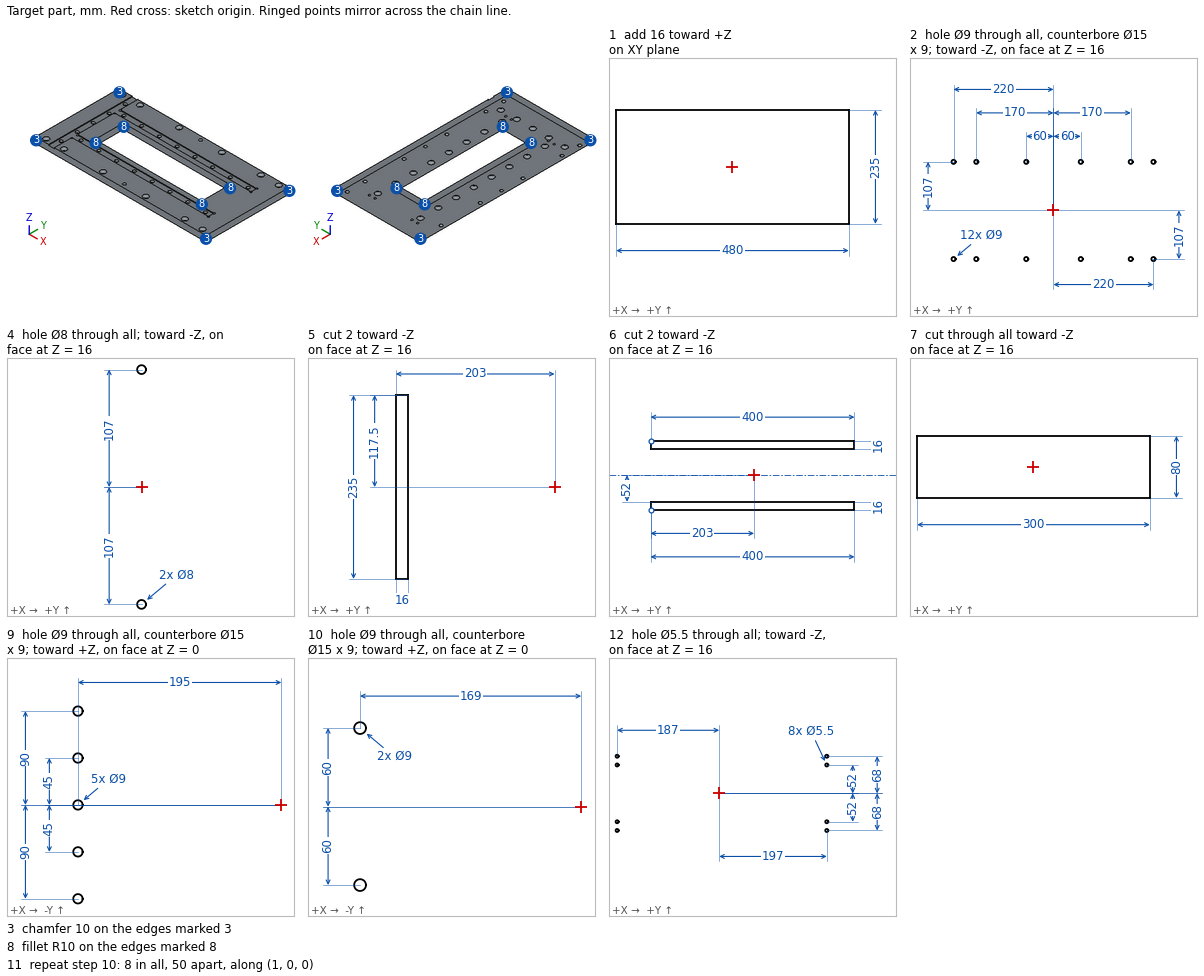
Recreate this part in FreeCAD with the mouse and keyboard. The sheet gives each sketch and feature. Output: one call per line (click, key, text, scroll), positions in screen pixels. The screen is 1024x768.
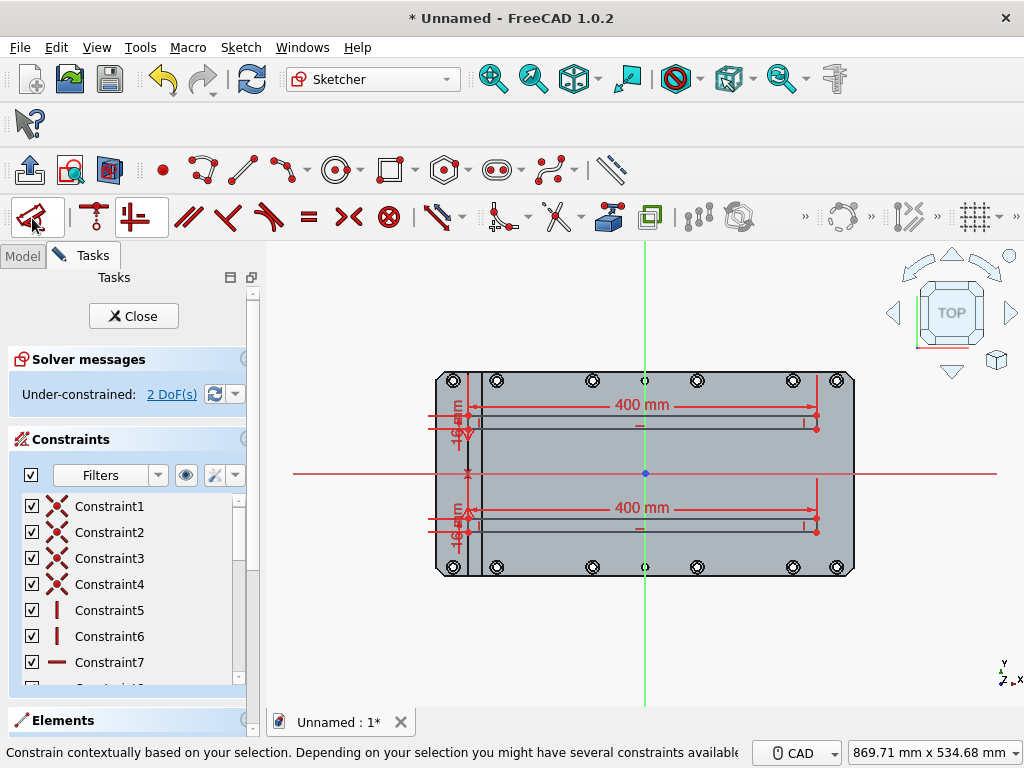
click(468, 519)
click(434, 496)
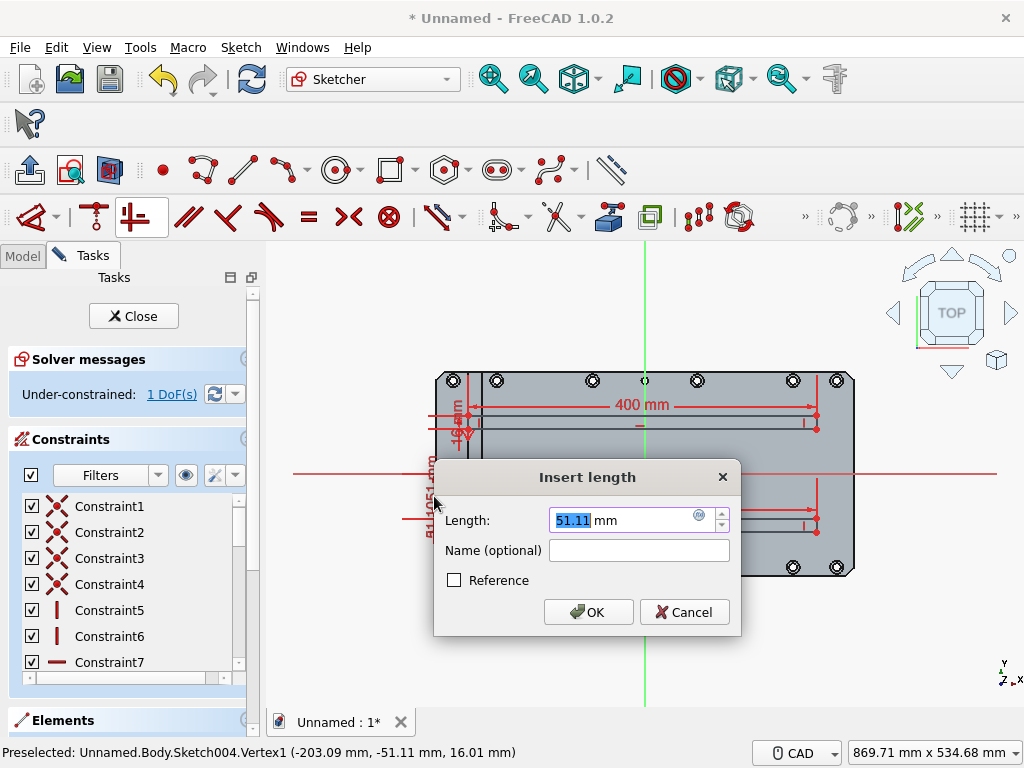
text(52)
key(Return)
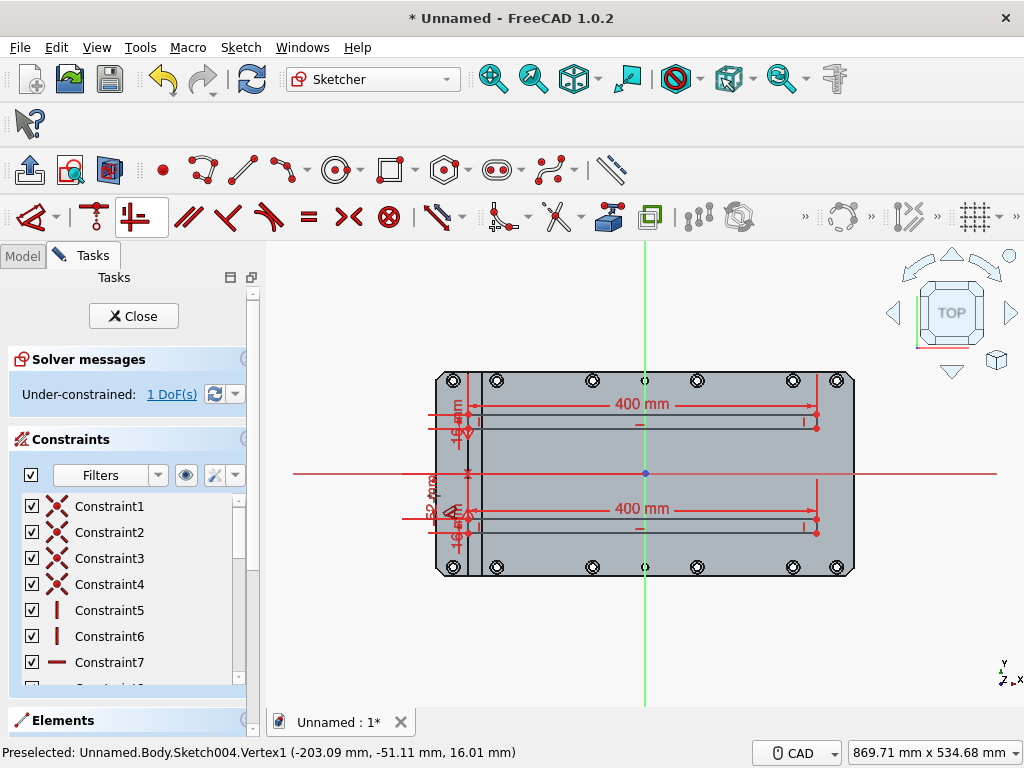
click(468, 519)
click(556, 553)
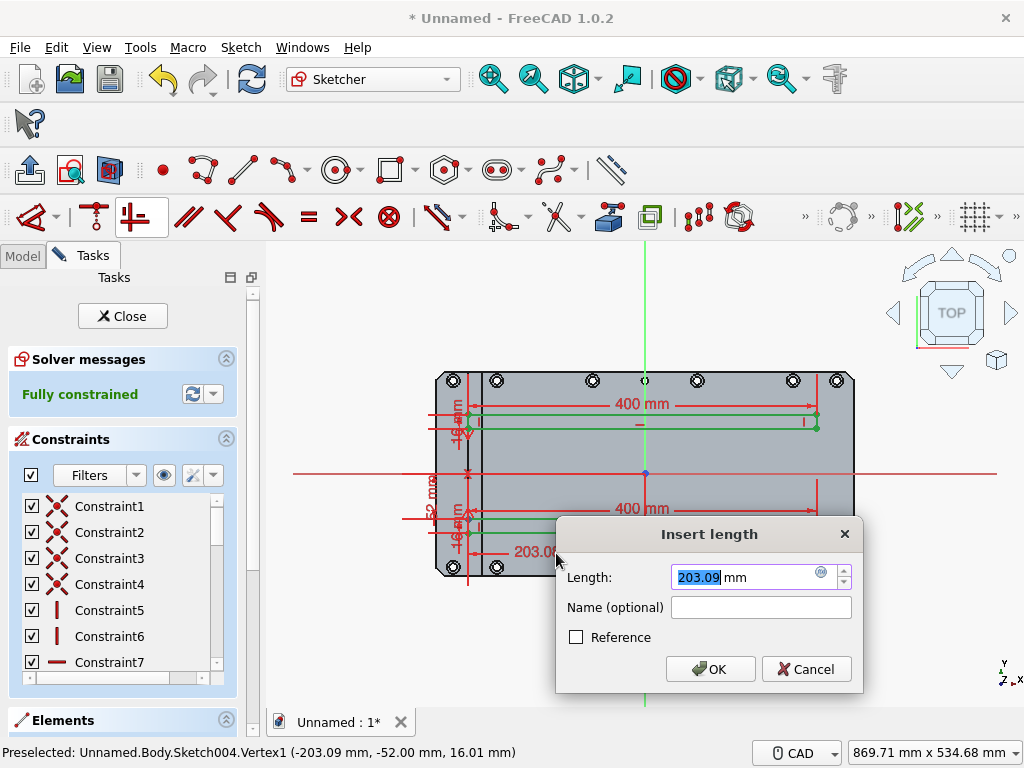
text(203)
key(Return)
key(Escape)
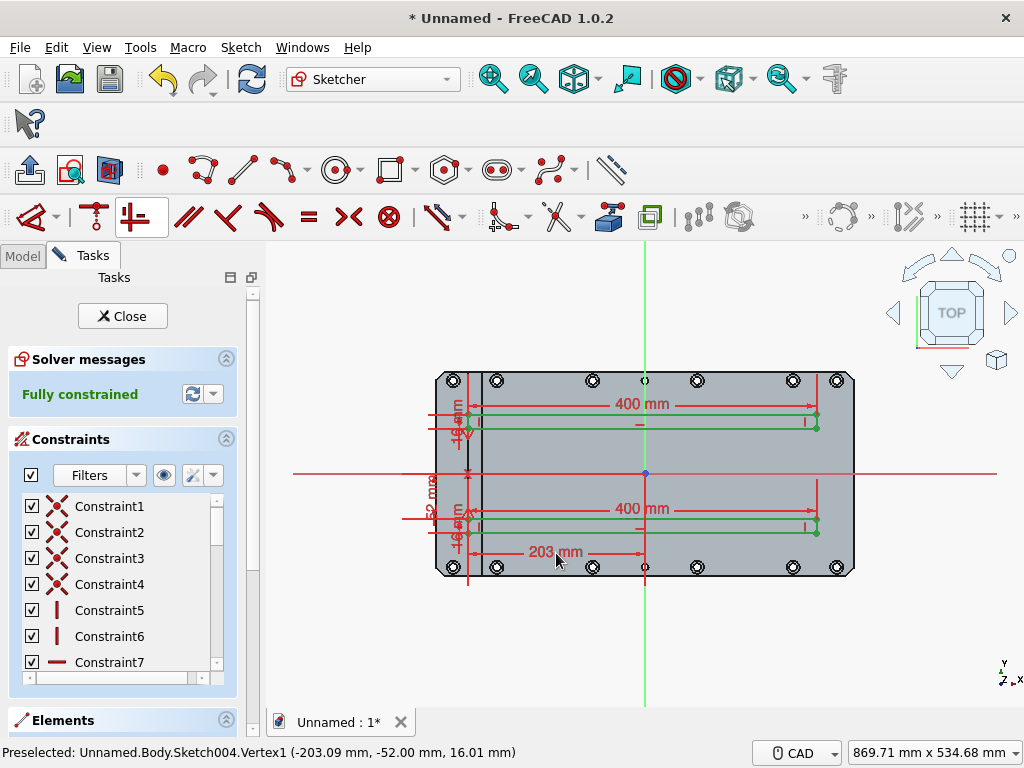
click(123, 316)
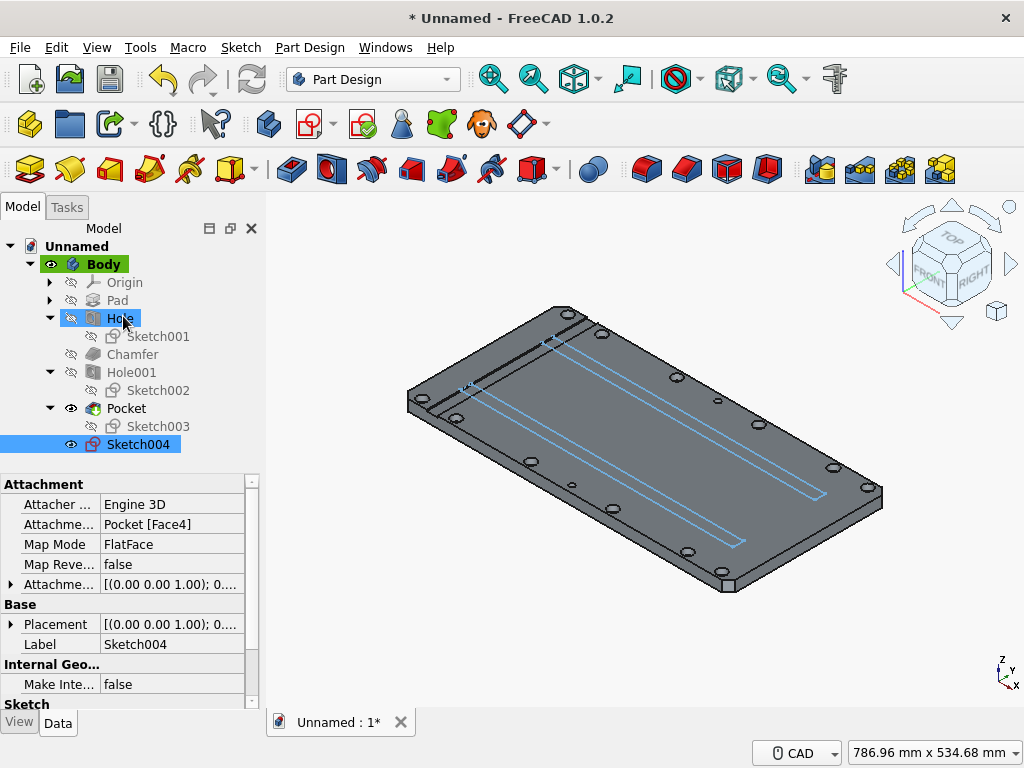
click(292, 170)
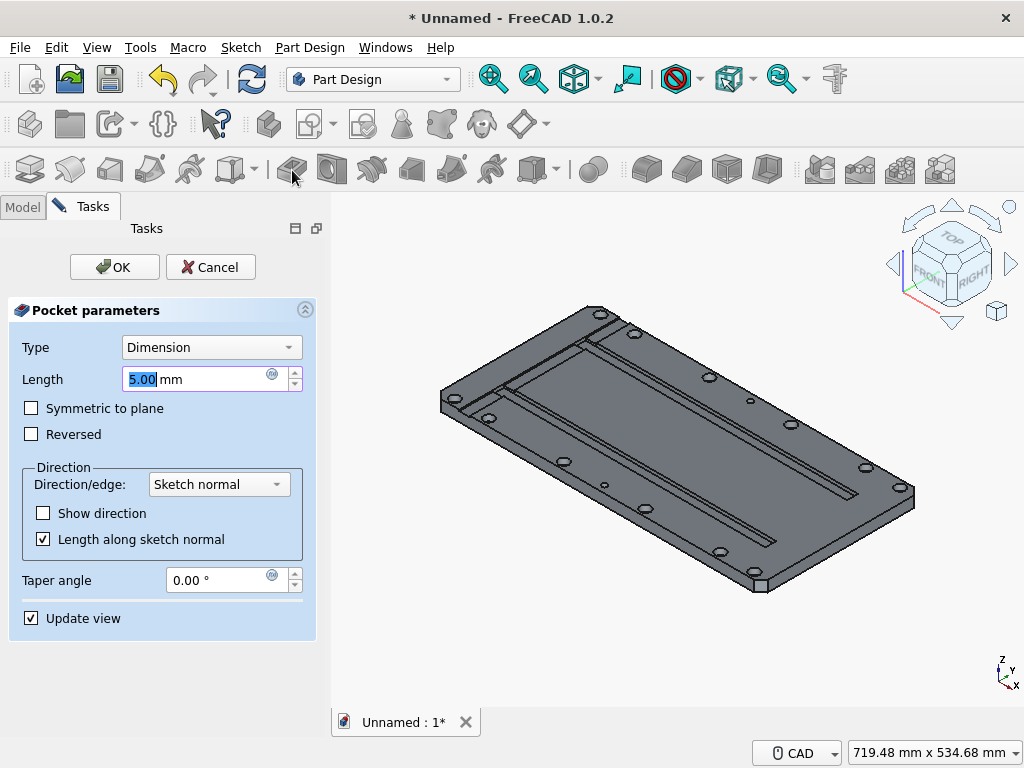
text(2)
key(Tab)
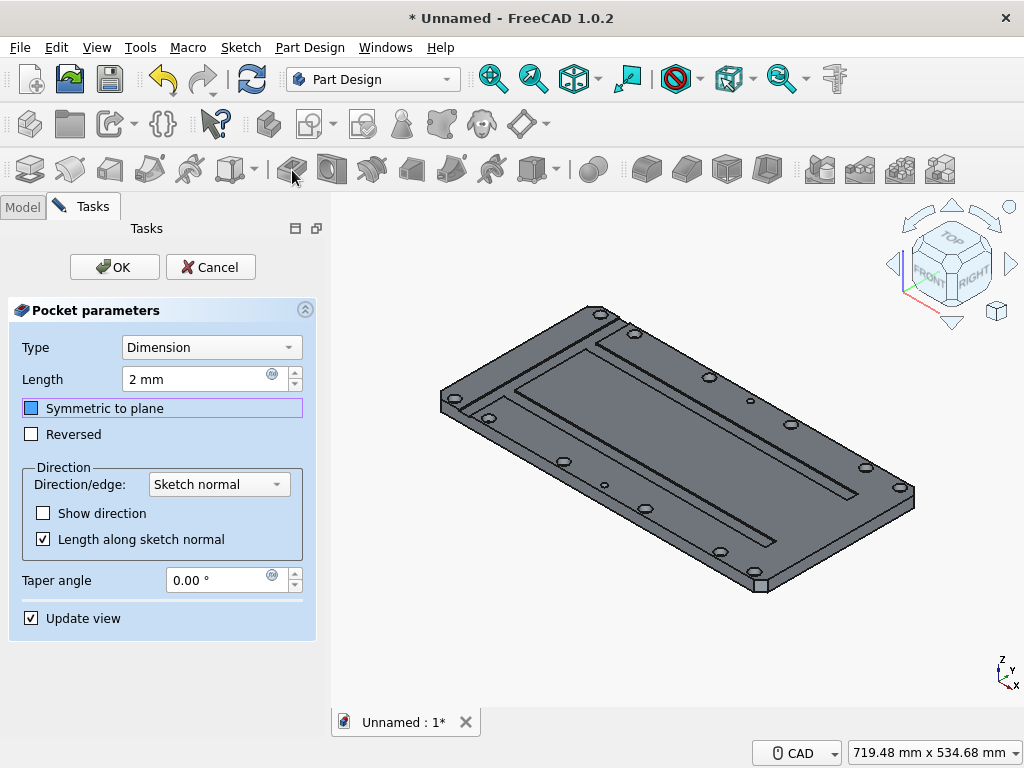
click(115, 267)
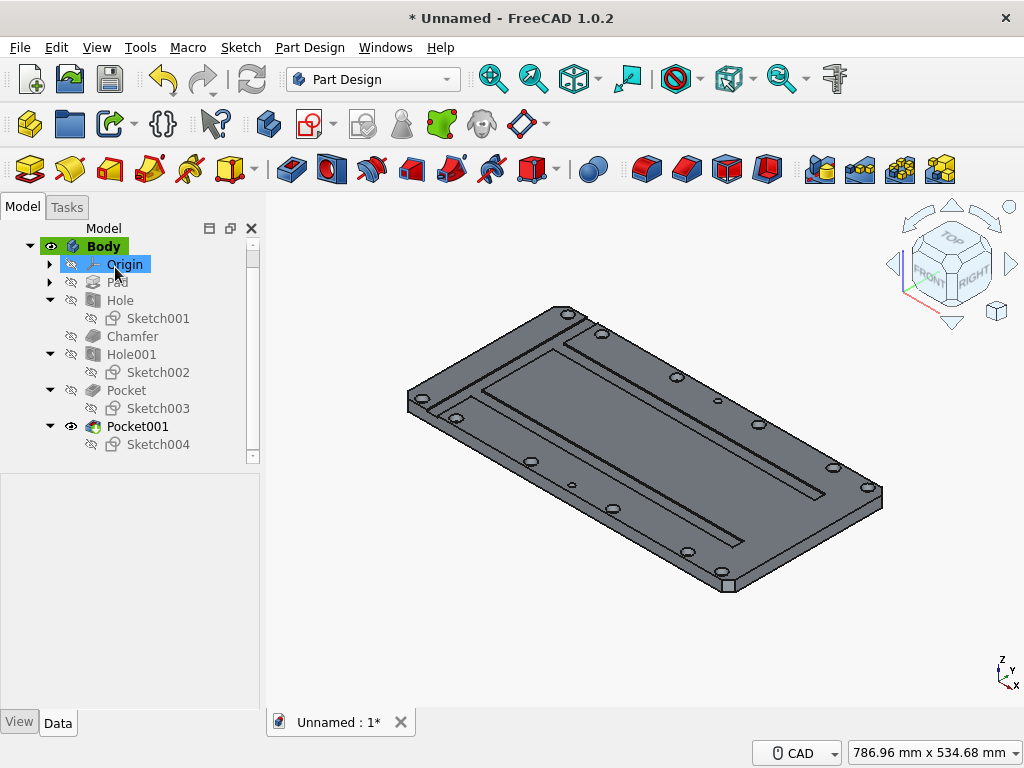
click(746, 501)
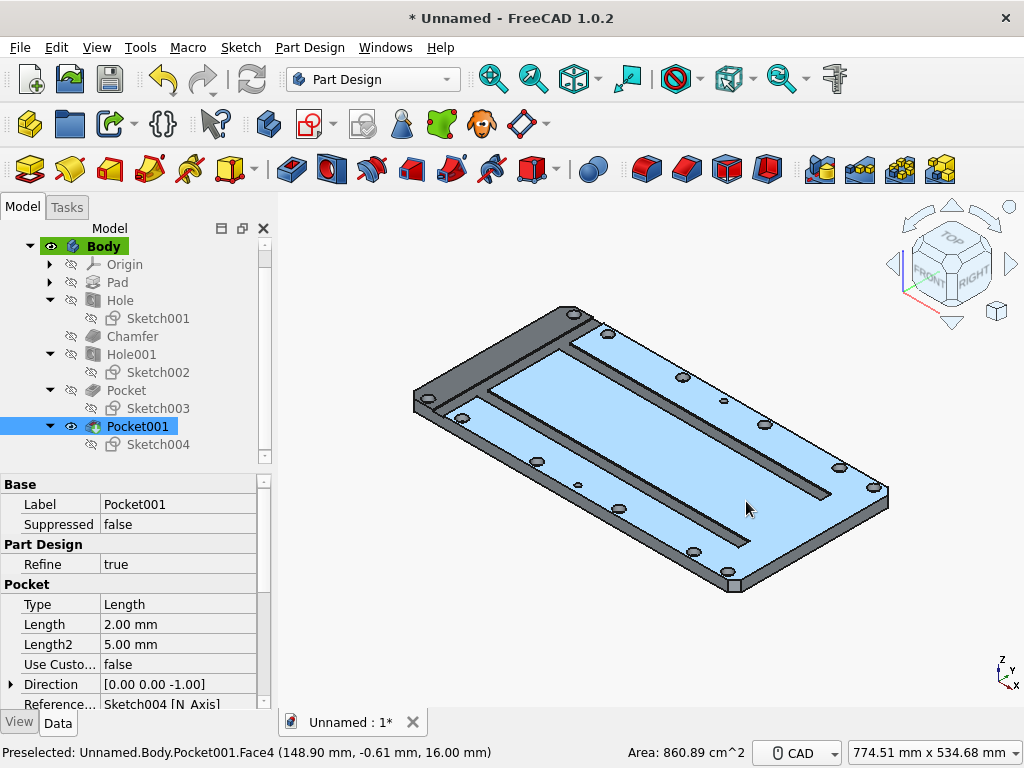
click(310, 124)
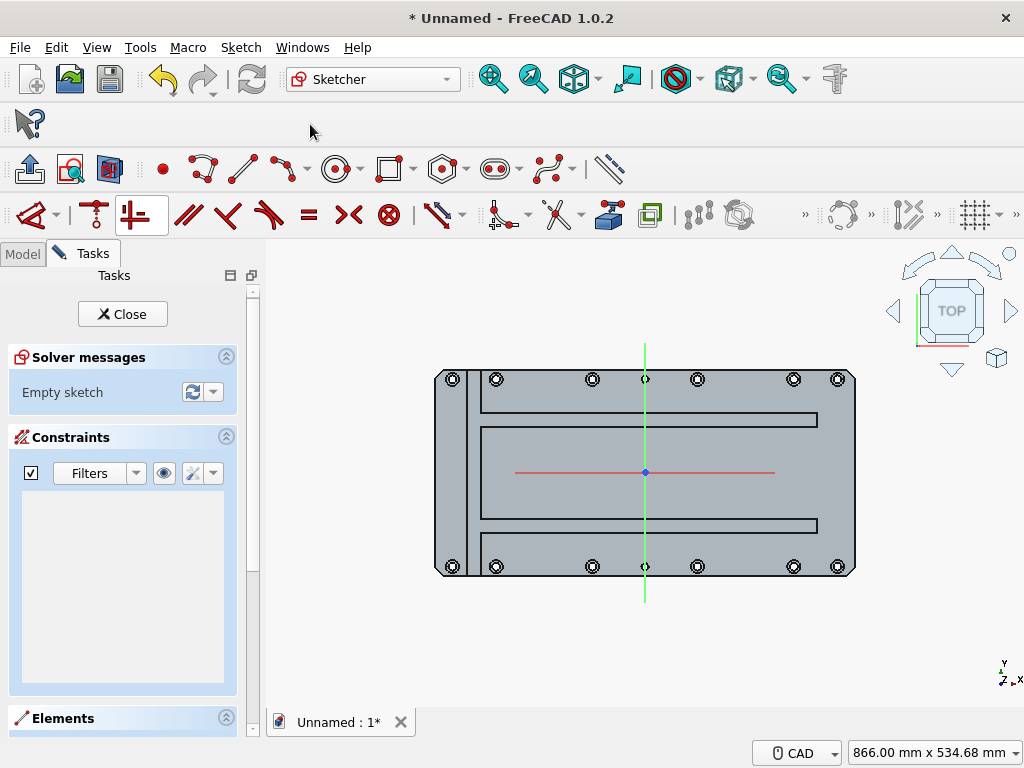
scroll(784, 473, up, 2)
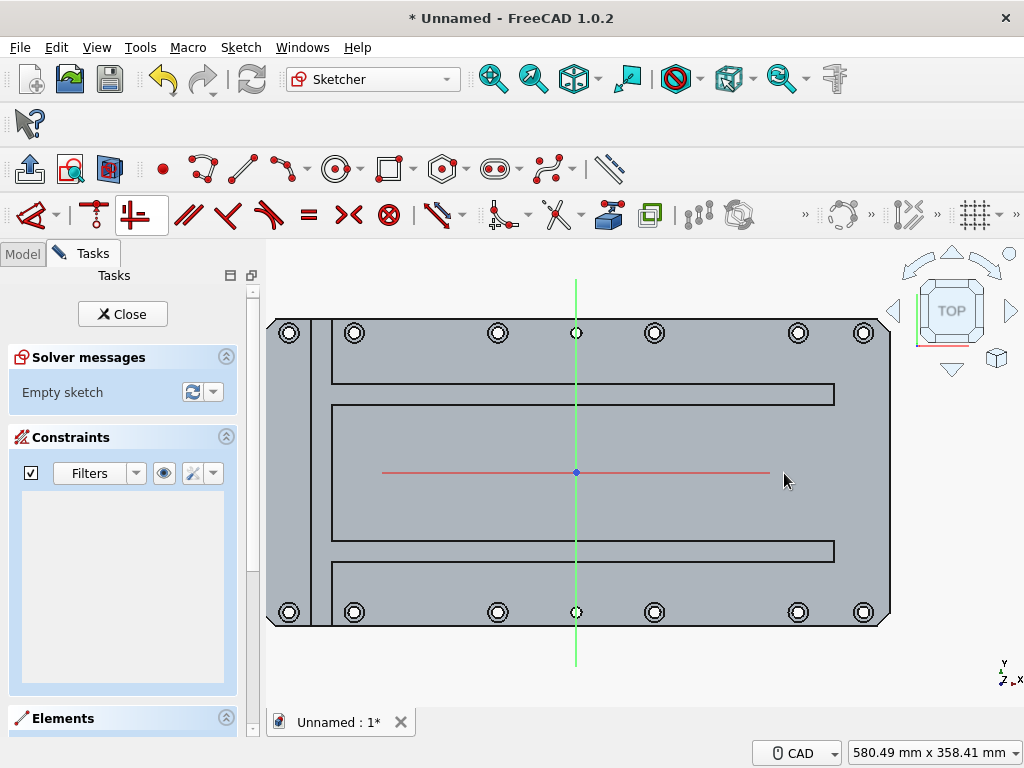
click(416, 170)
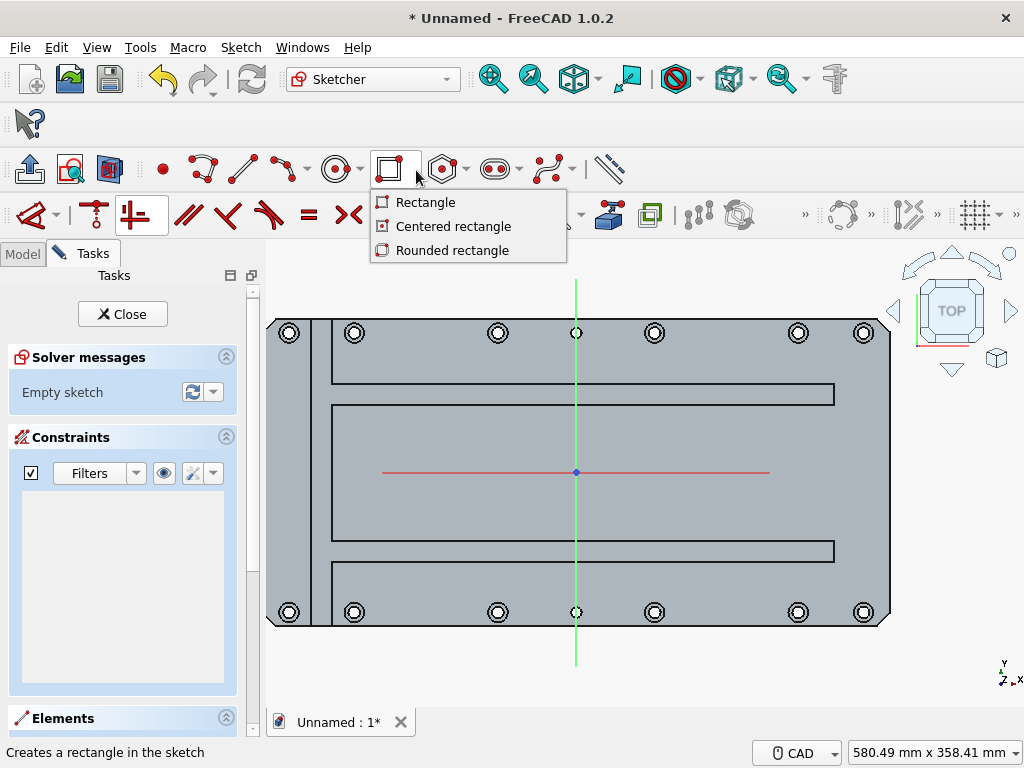
click(468, 226)